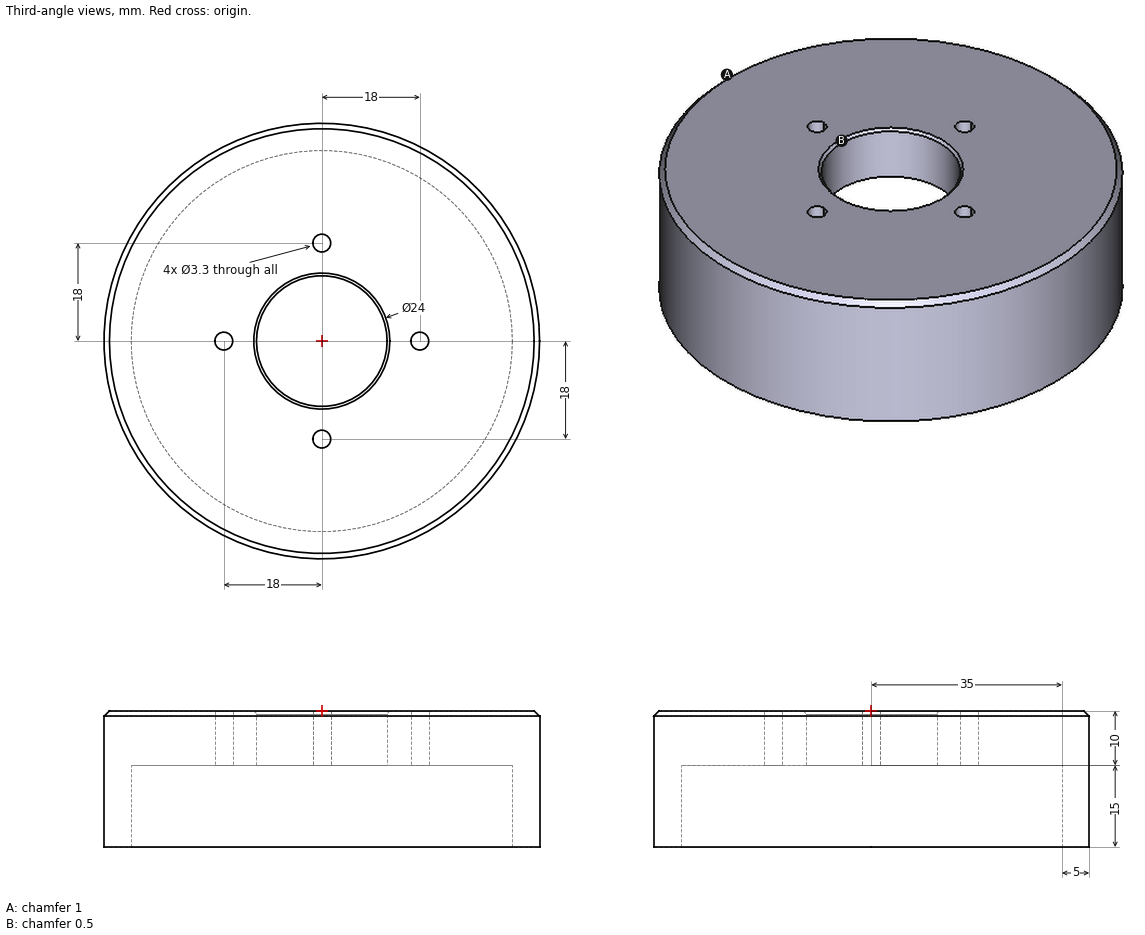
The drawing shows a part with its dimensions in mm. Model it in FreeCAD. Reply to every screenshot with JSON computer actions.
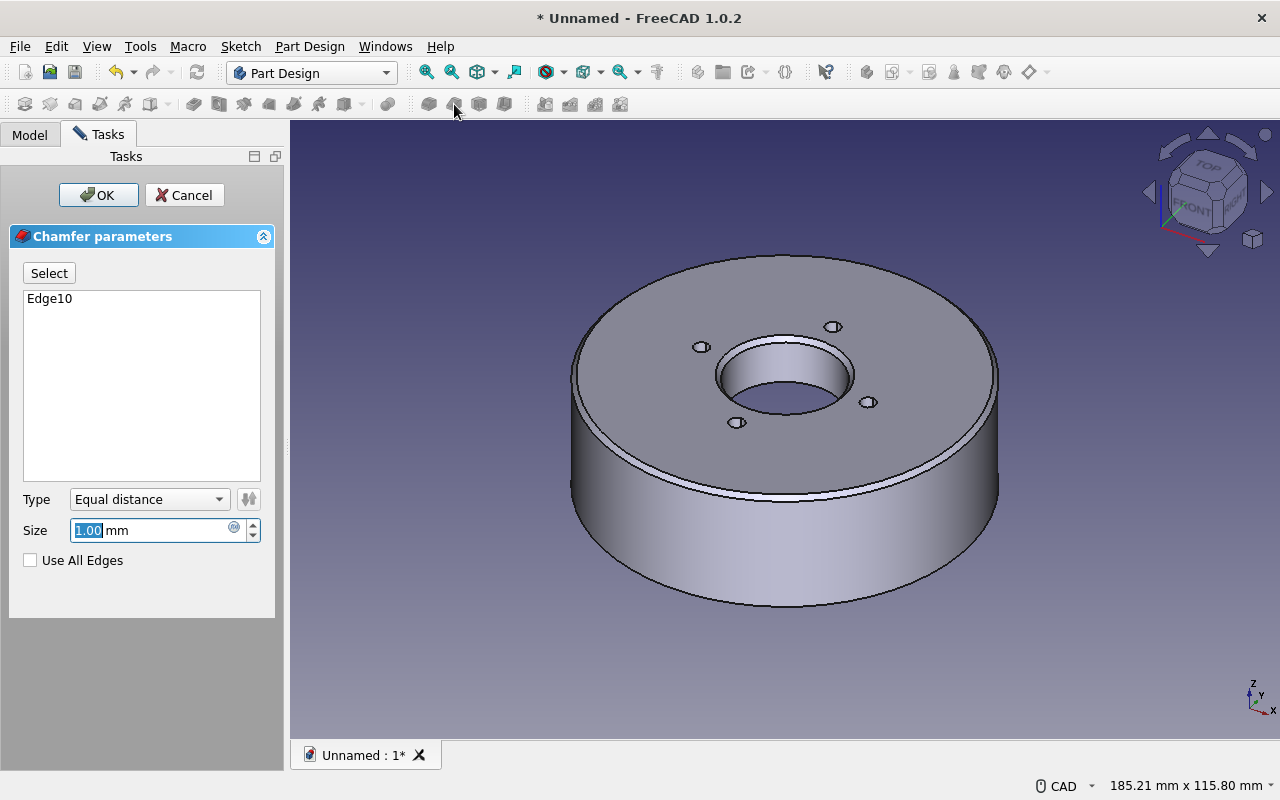
{"action": "type", "text": "0.5"}
{"action": "key", "text": "Tab"}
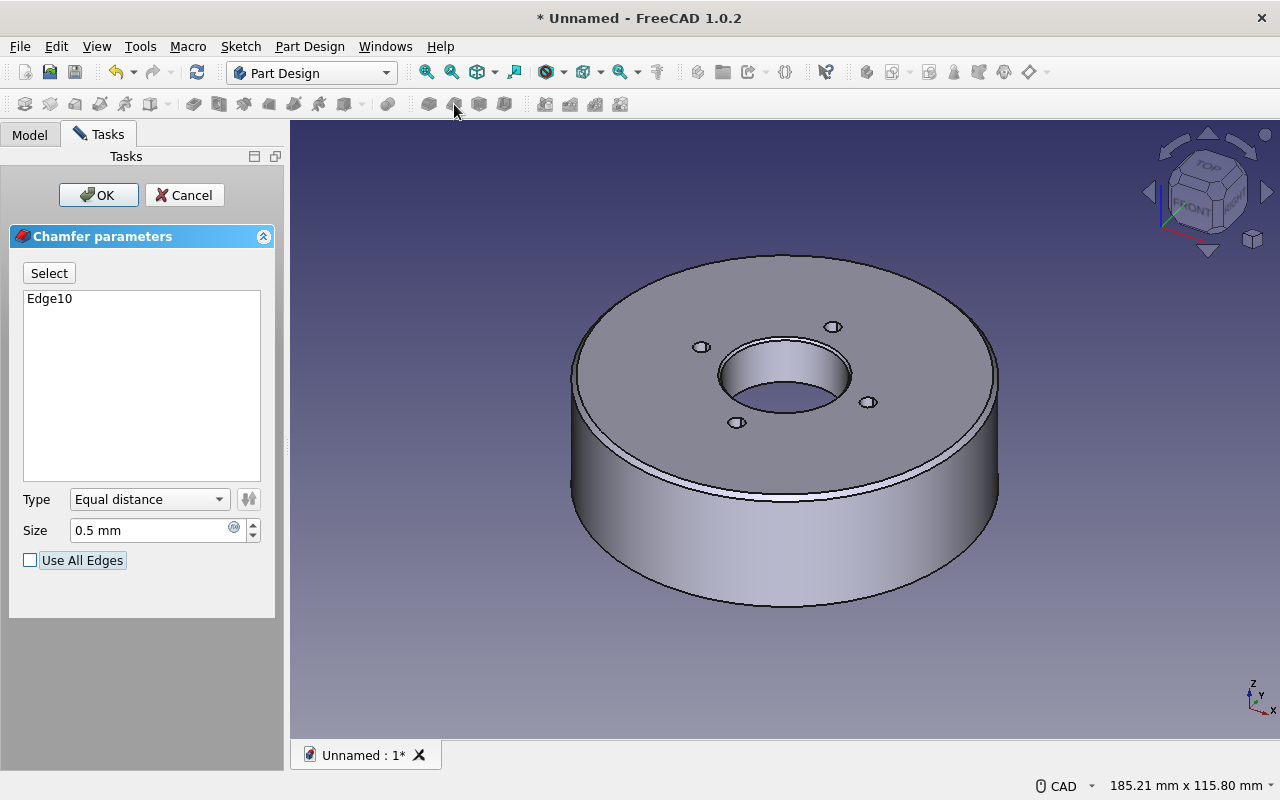
{"action": "left_click", "coordinate": [99, 195]}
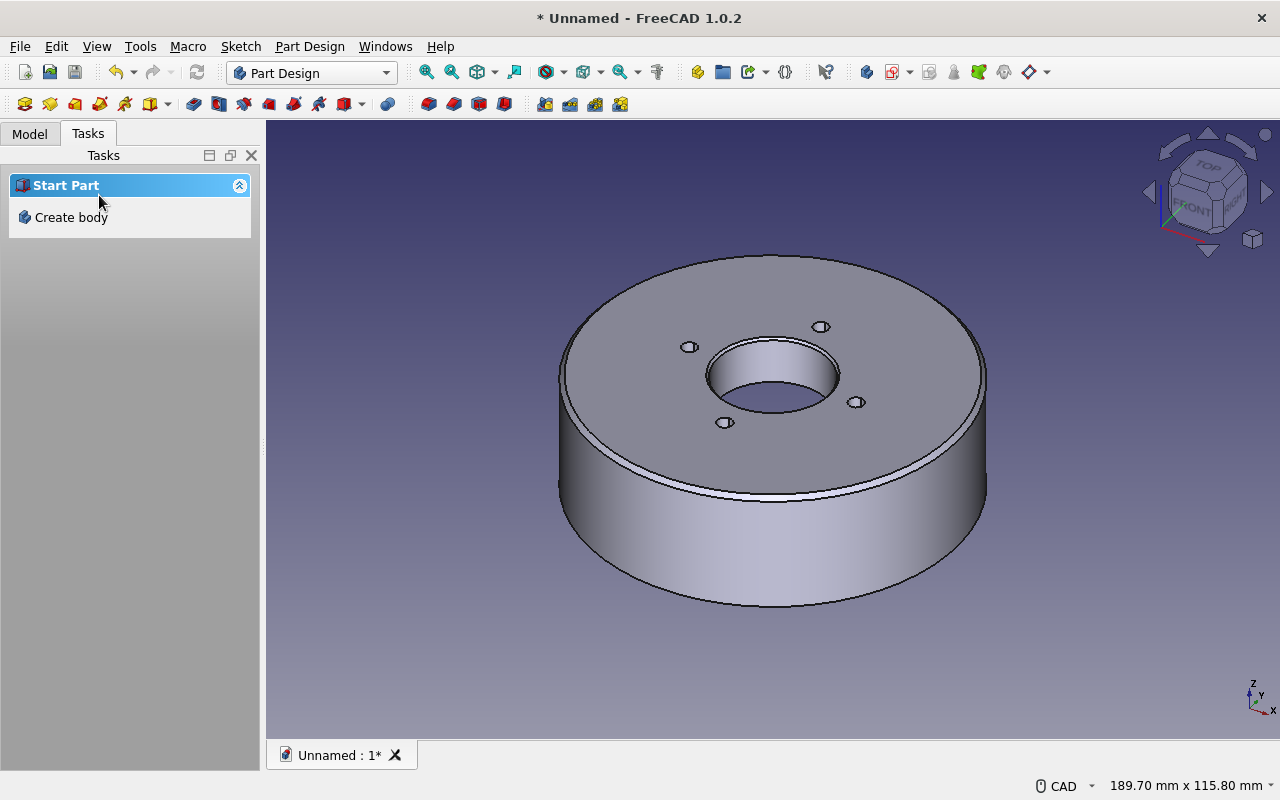
{"action": "key", "text": "0"}